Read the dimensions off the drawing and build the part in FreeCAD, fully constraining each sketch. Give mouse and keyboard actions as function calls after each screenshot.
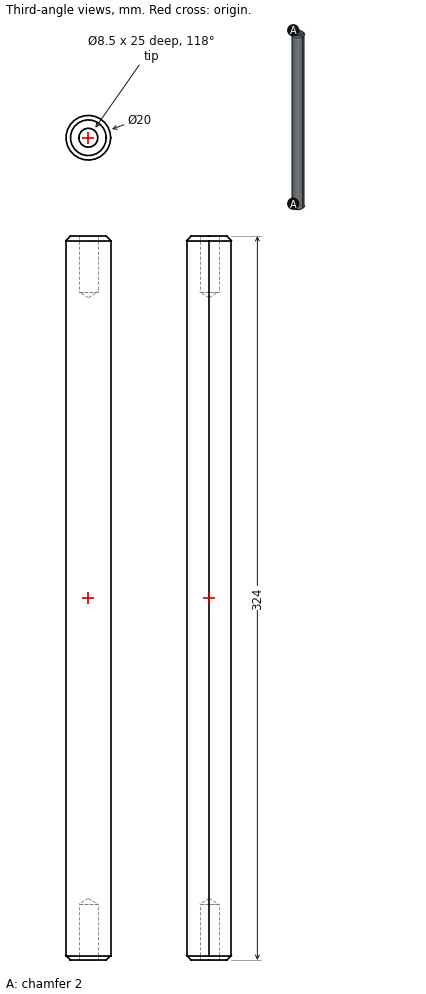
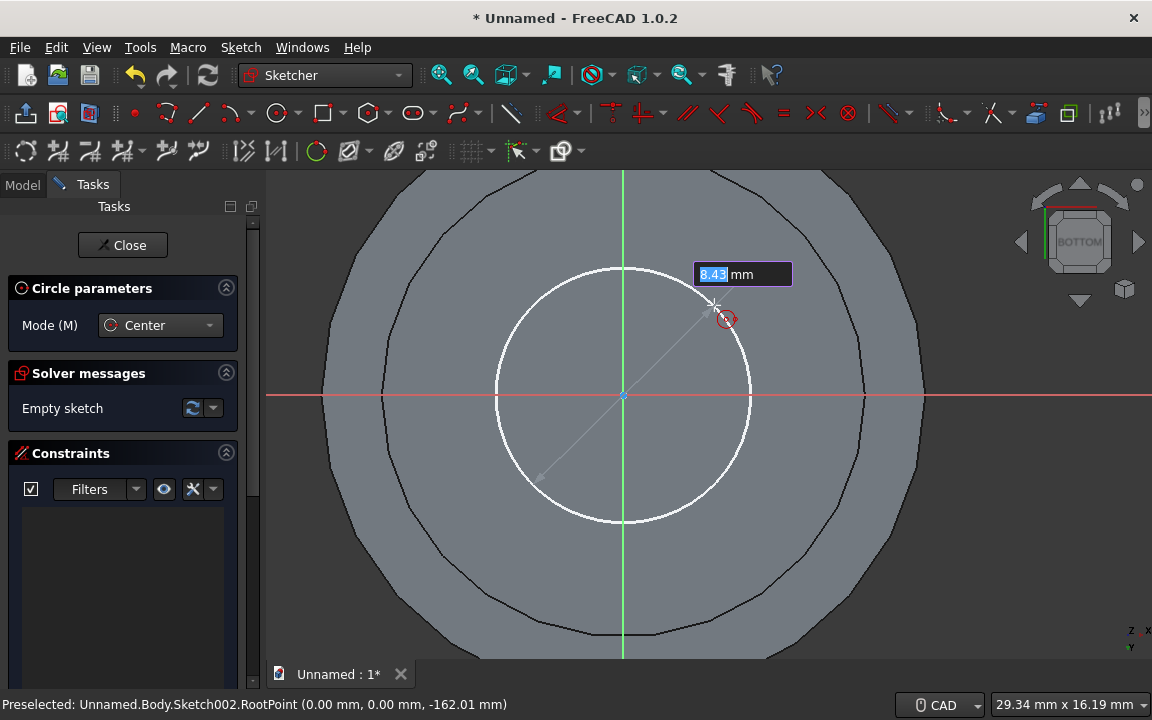
text(8.5)
key(Return)
key(Escape)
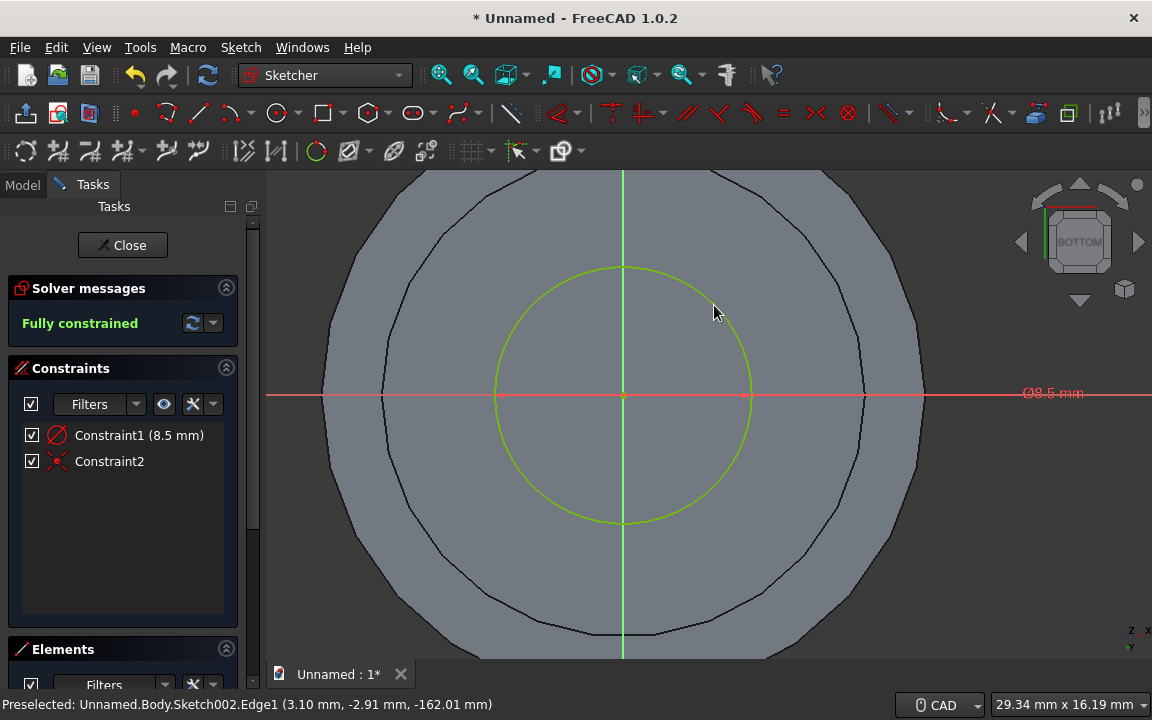
click(123, 245)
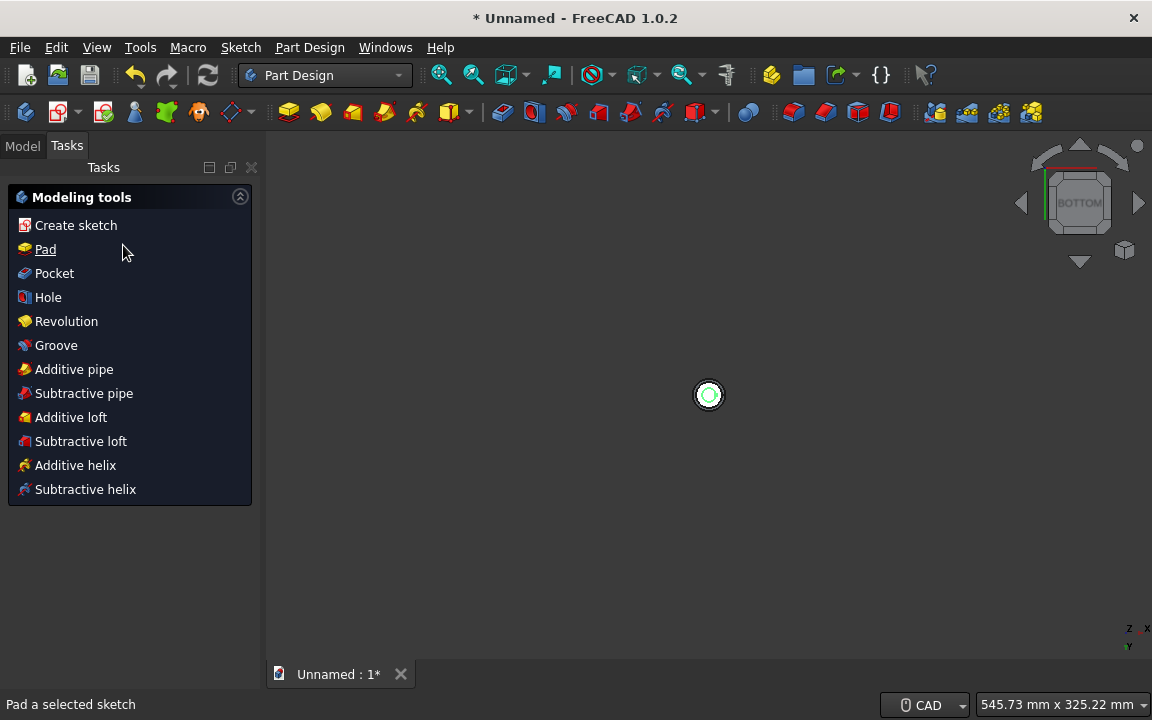
click(536, 112)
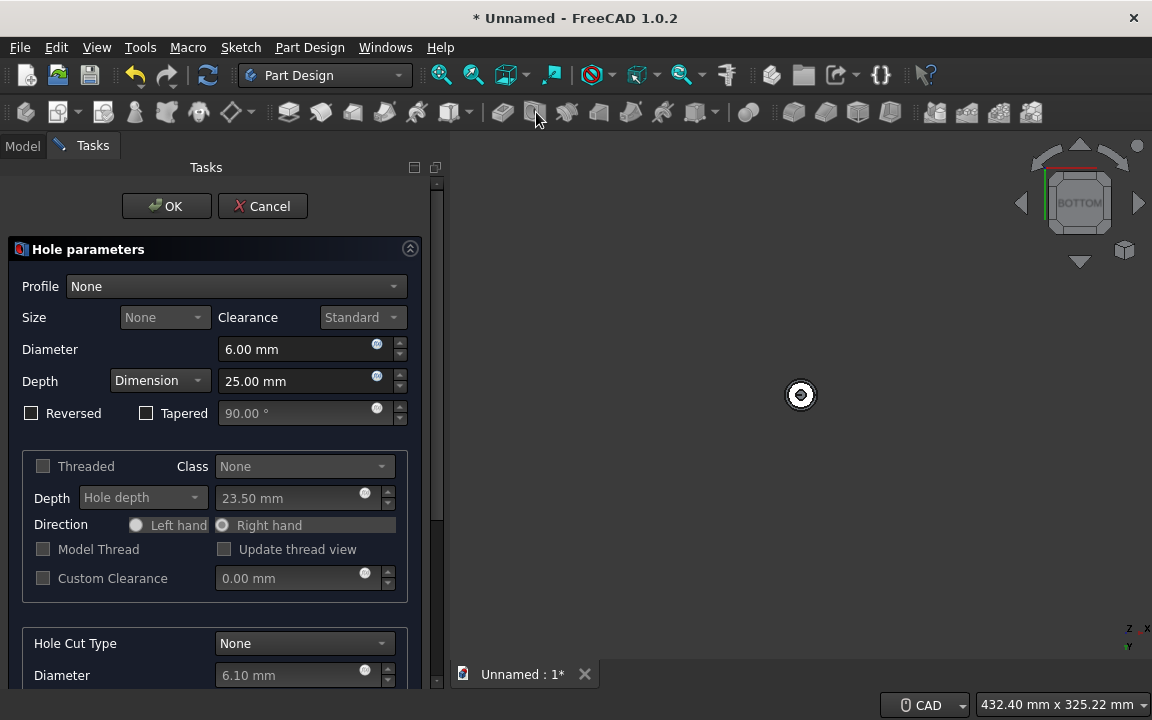
triple_click(305, 349)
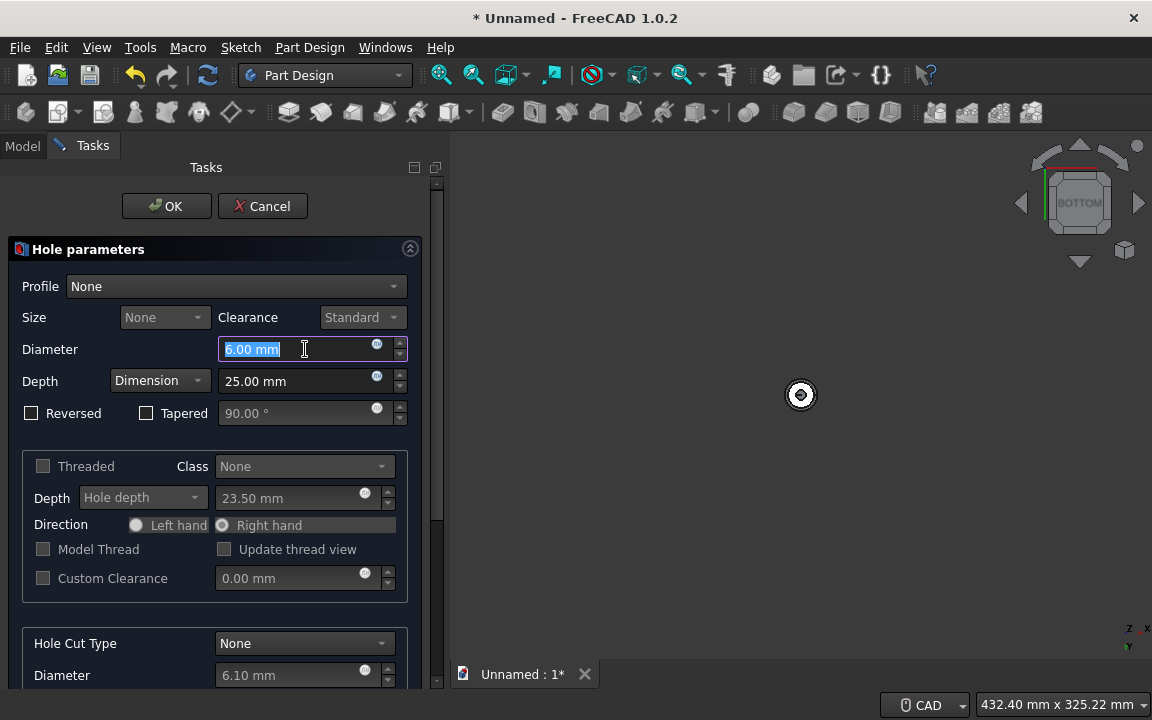
text(8.5)
key(Tab)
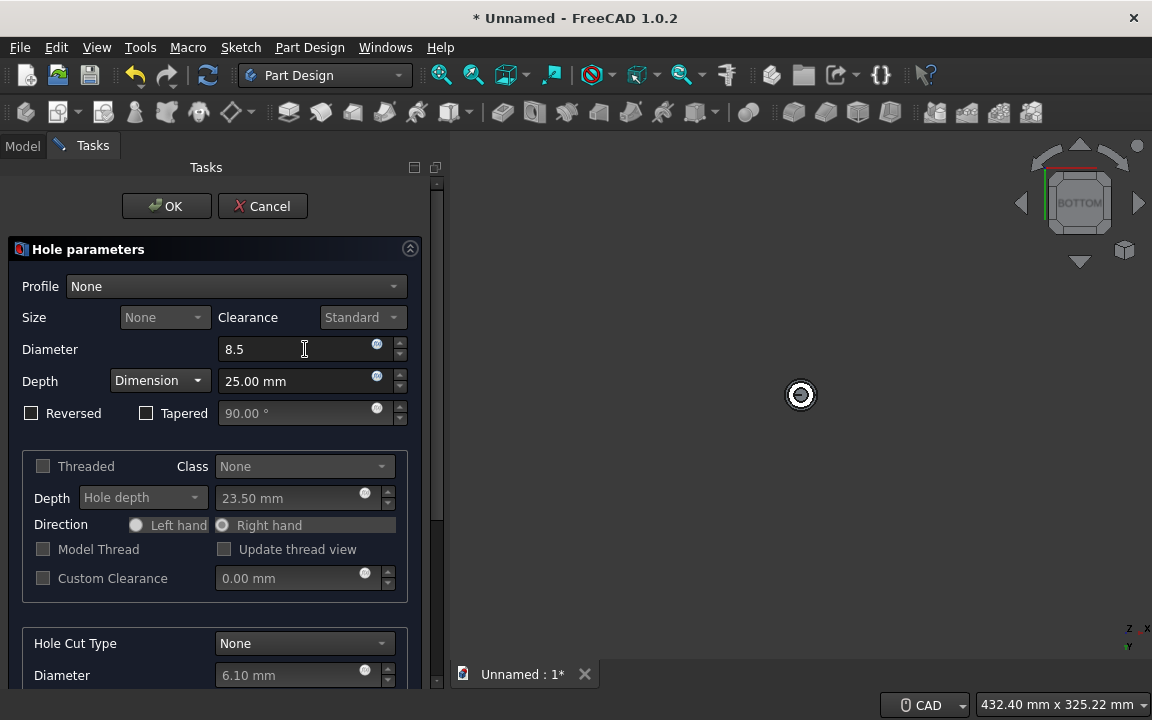
triple_click(305, 381)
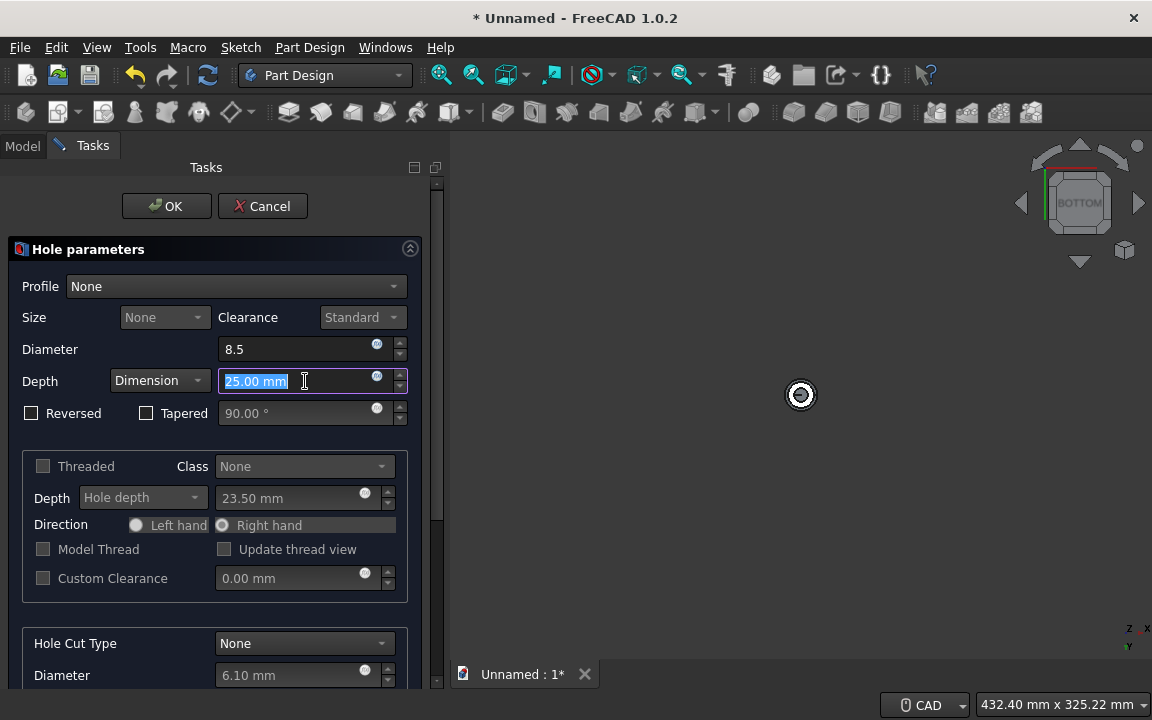
text(25)
key(Tab)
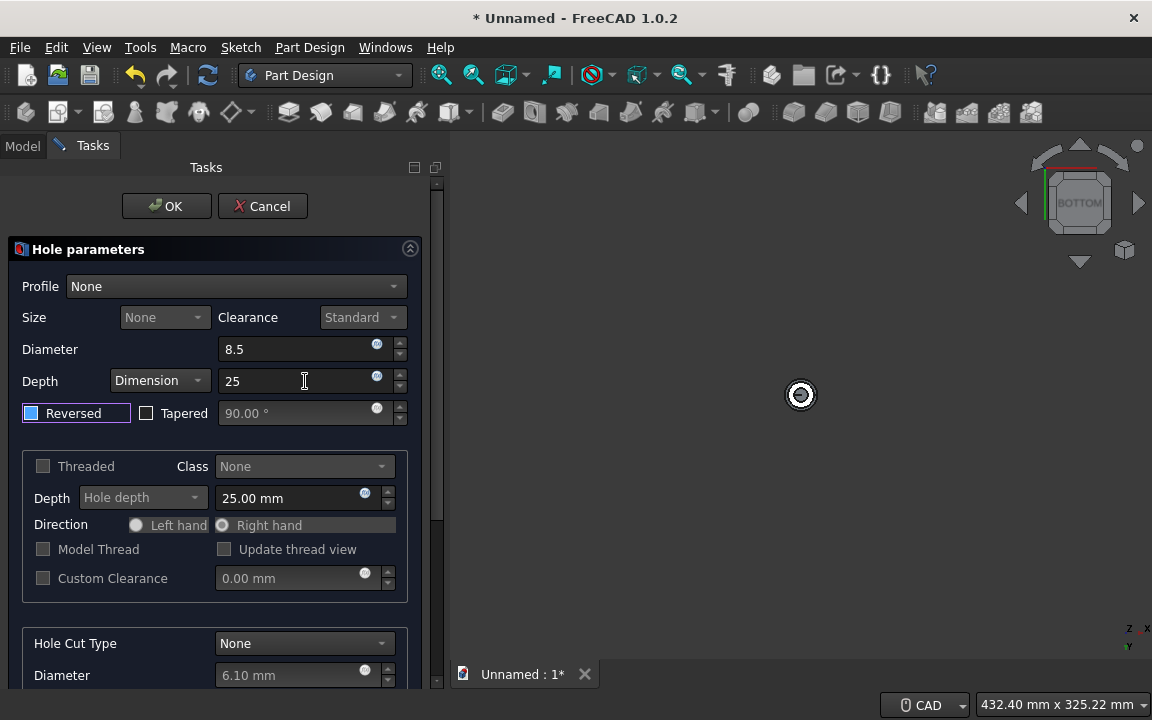
click(167, 206)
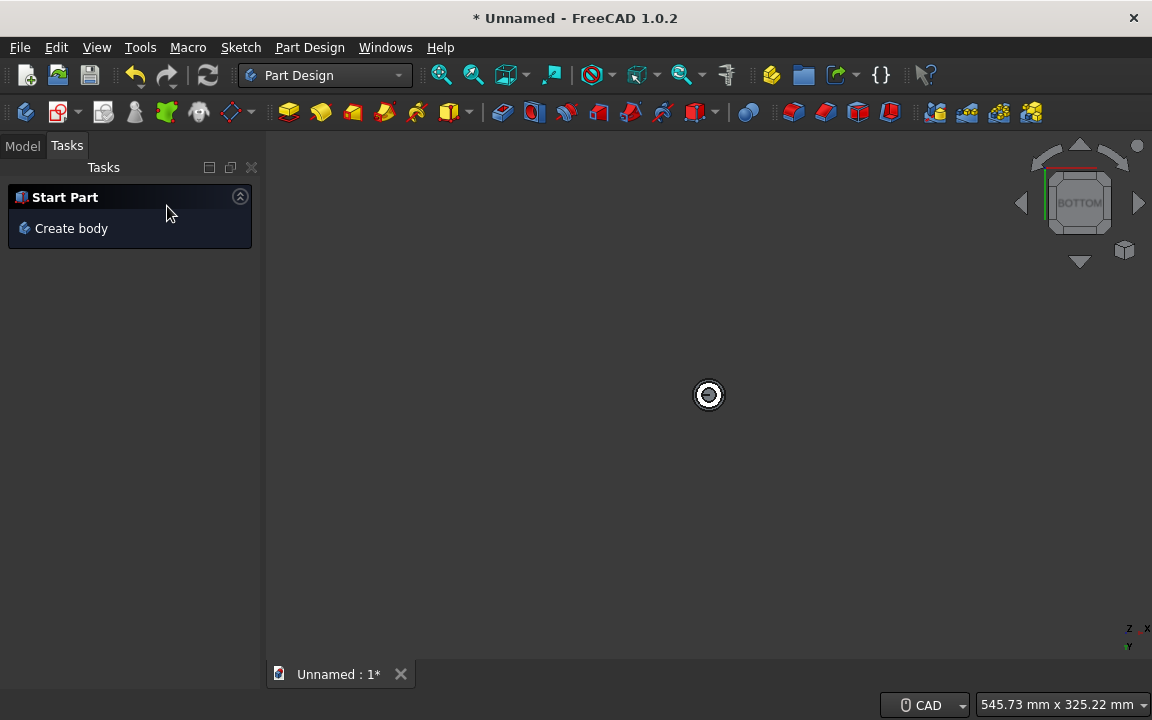
key(0)